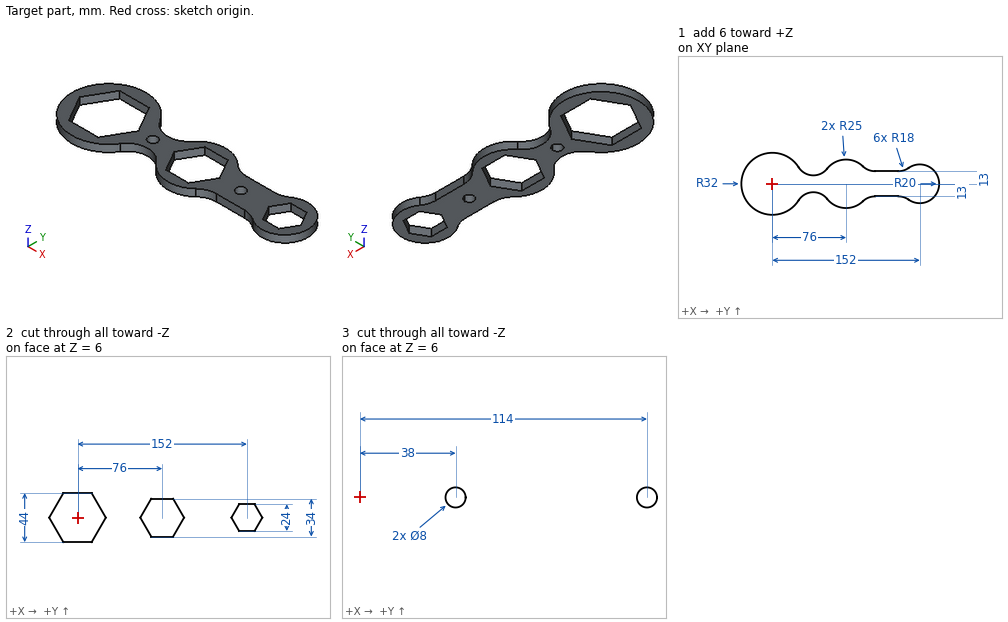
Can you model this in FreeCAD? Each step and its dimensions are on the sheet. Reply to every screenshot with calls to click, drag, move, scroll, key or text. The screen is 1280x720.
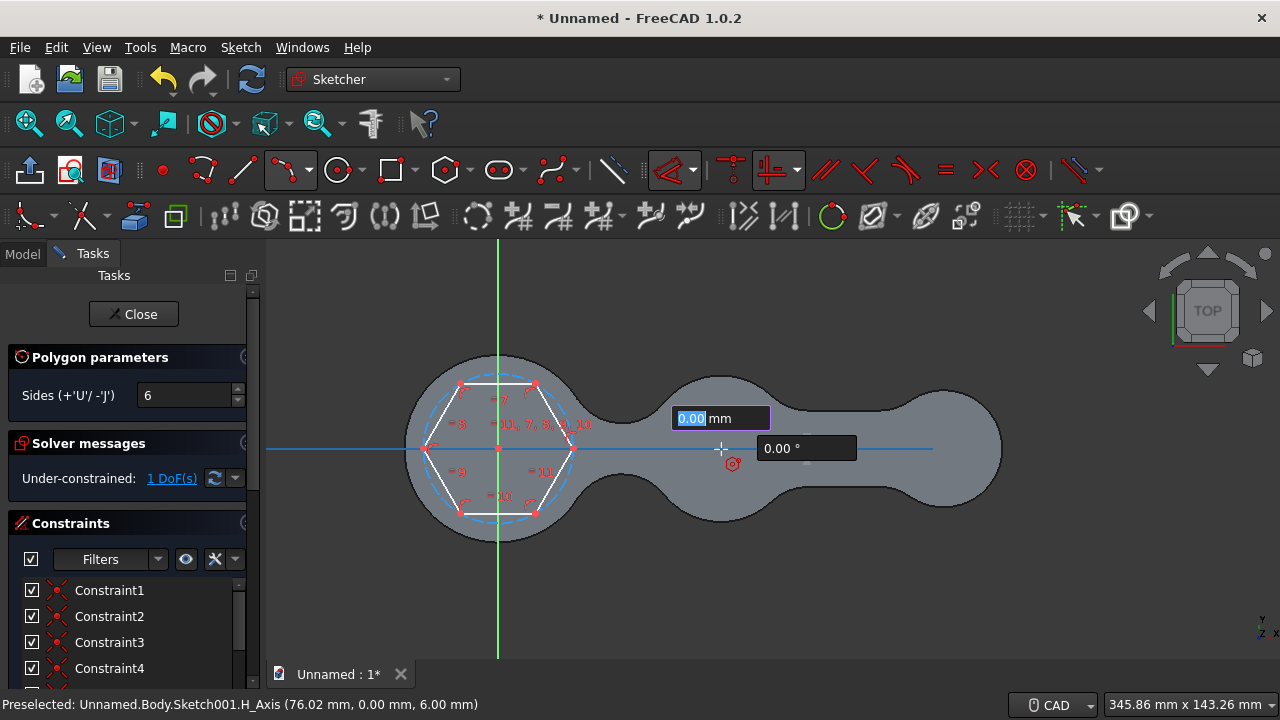
click(778, 449)
key(Escape)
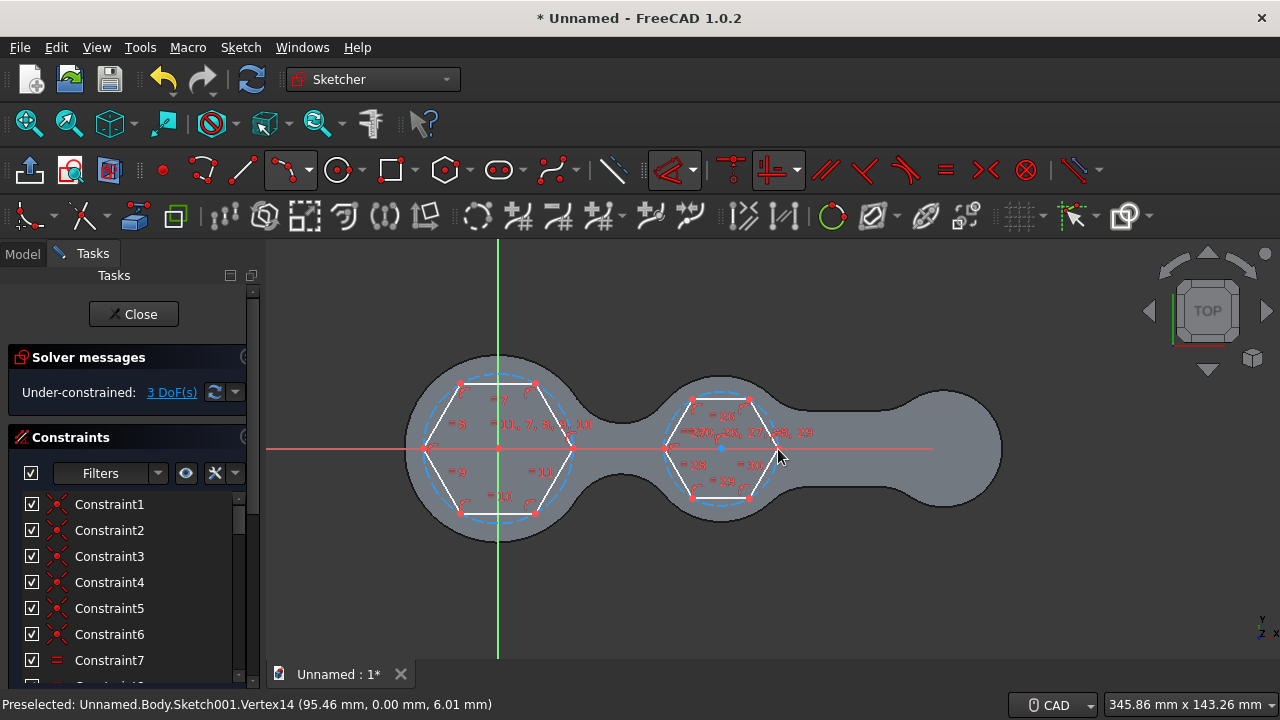
click(446, 170)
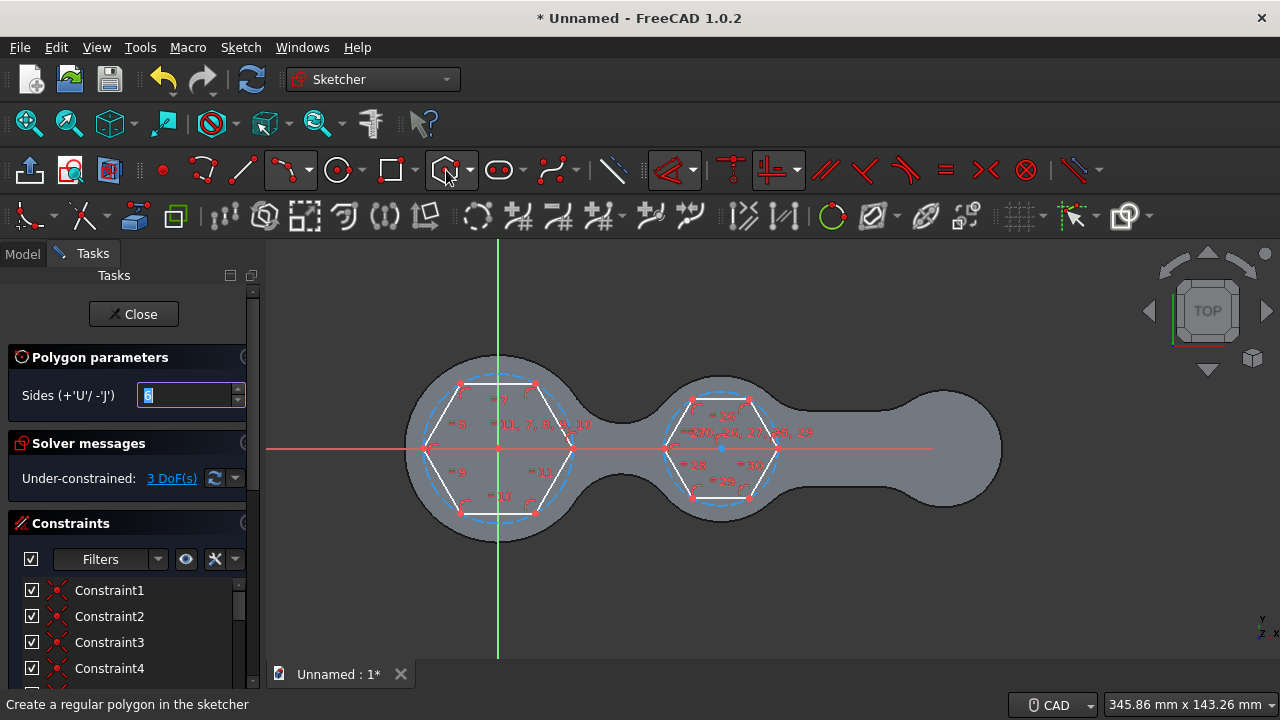
click(944, 449)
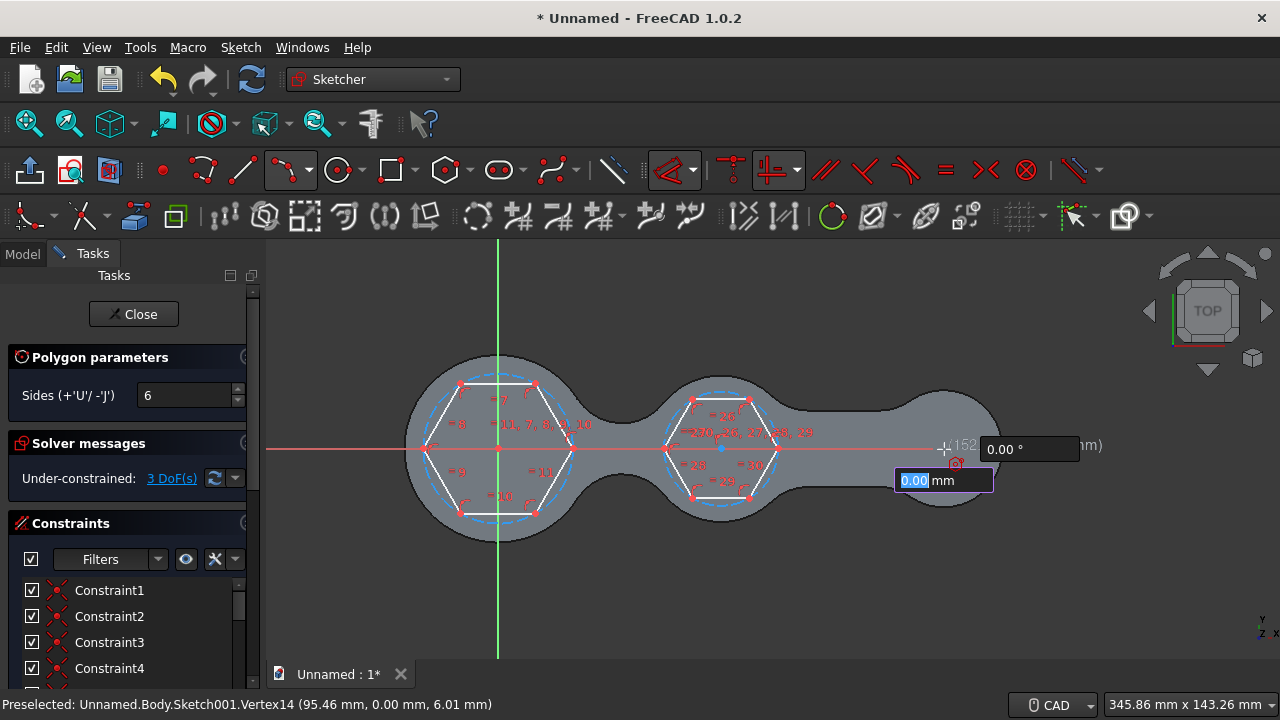
click(984, 449)
key(Escape)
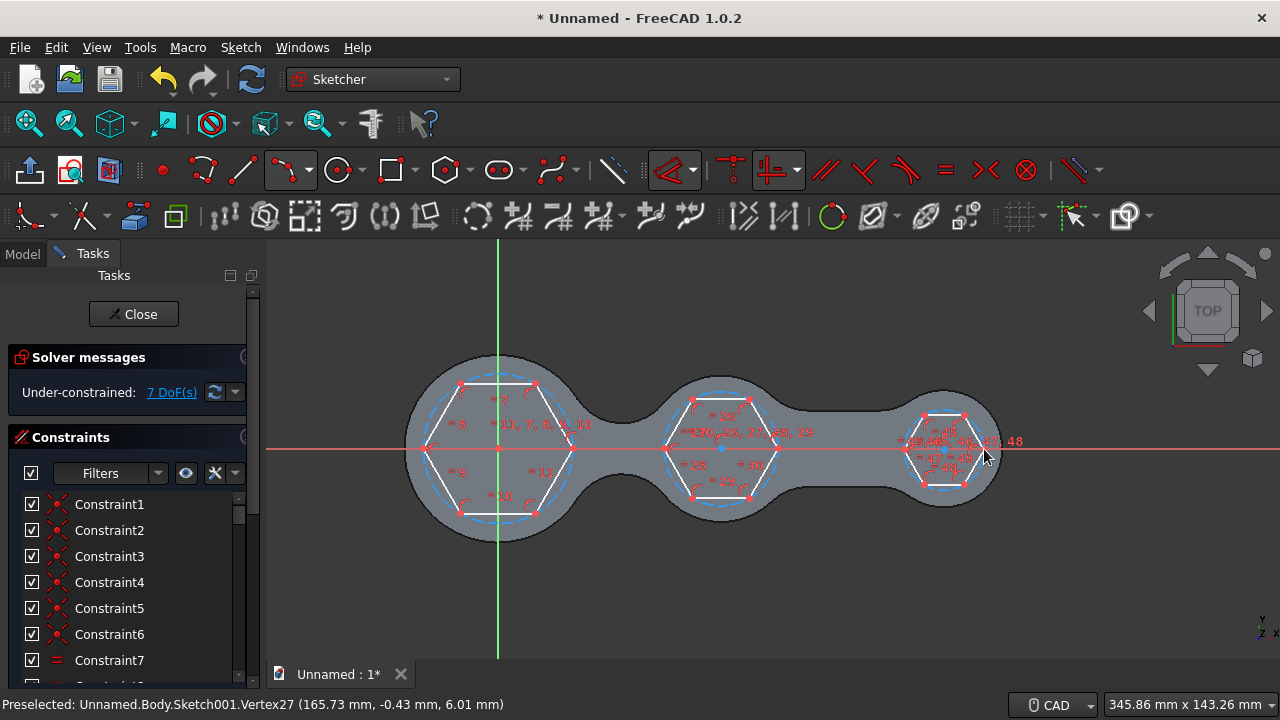
scroll(944, 415, up, 5)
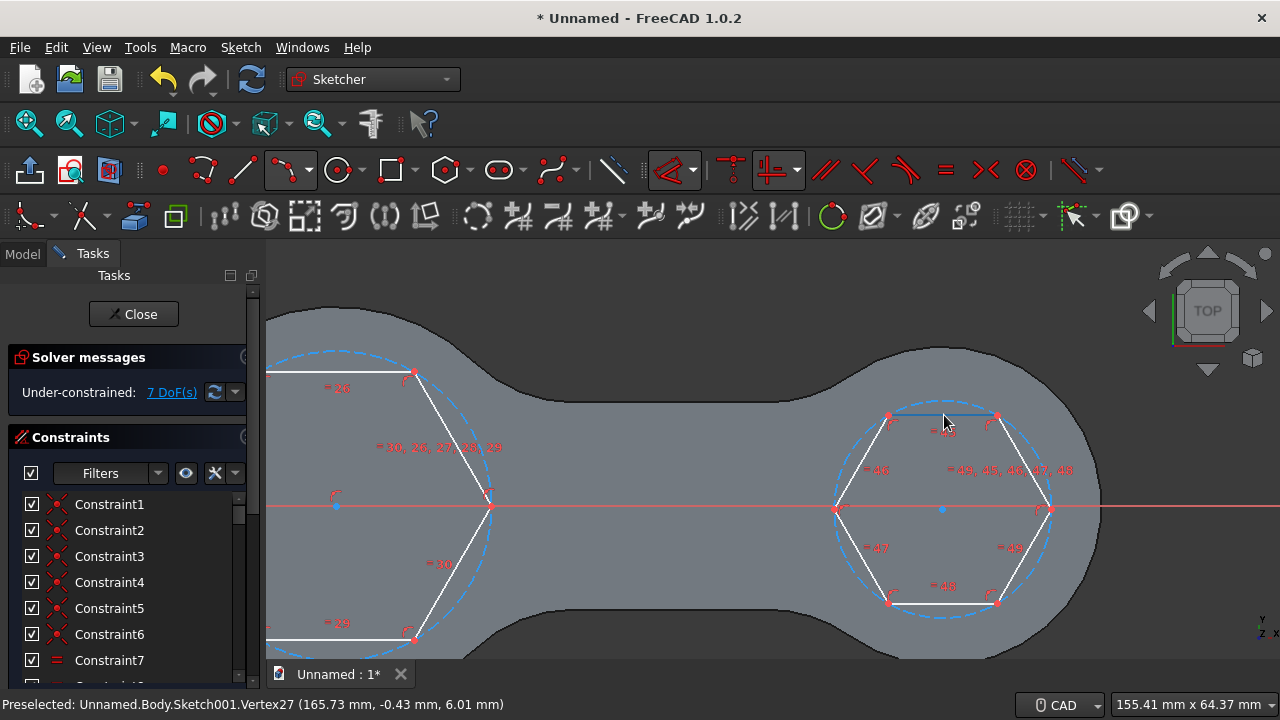
click(943, 415)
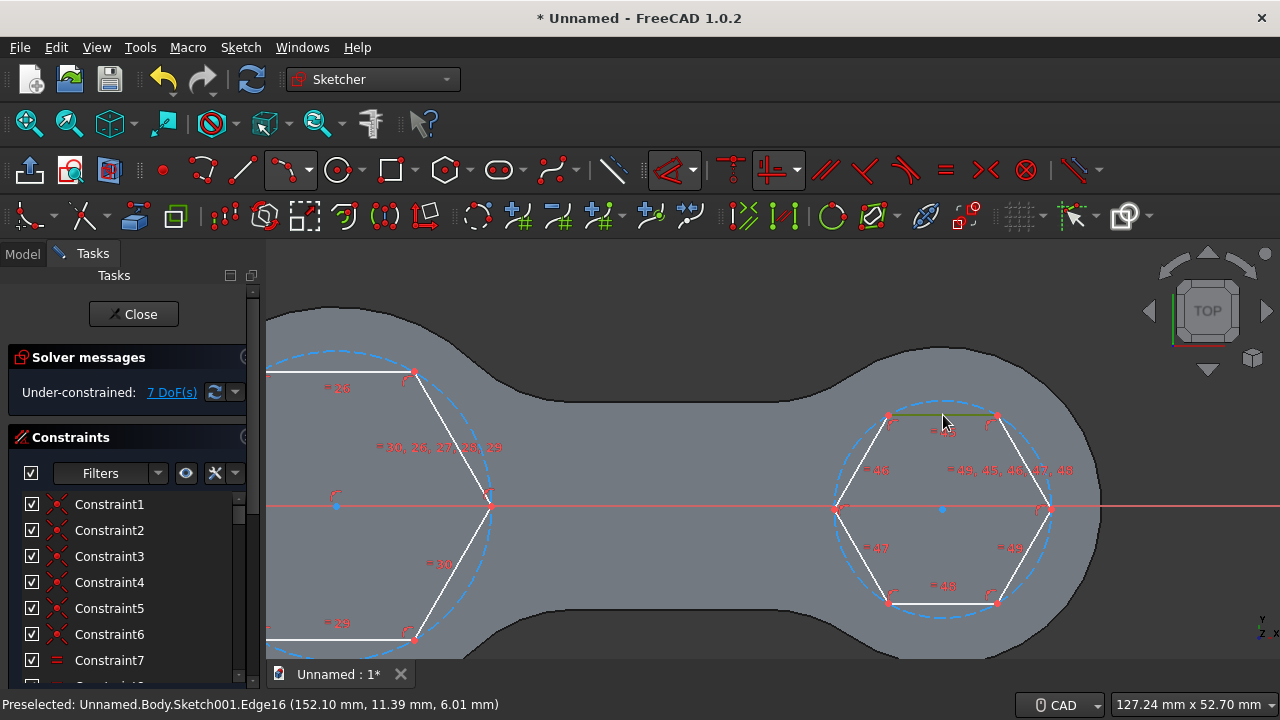
key(h)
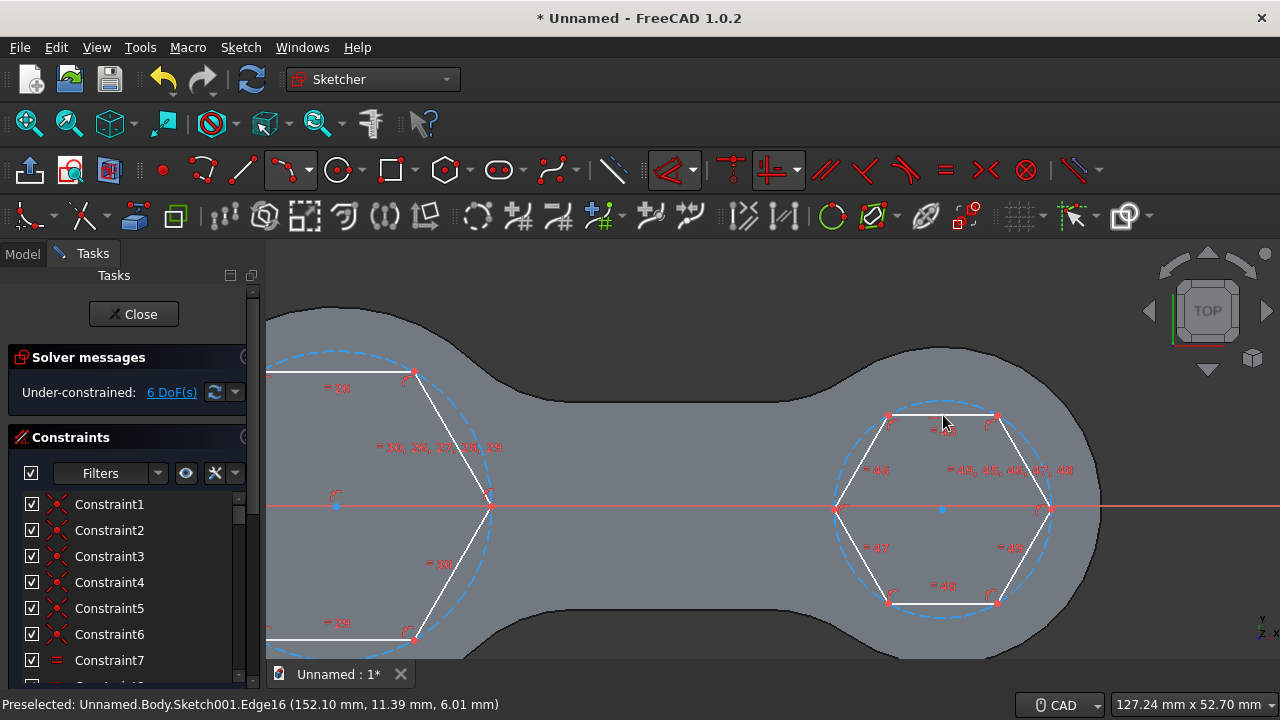
click(943, 509)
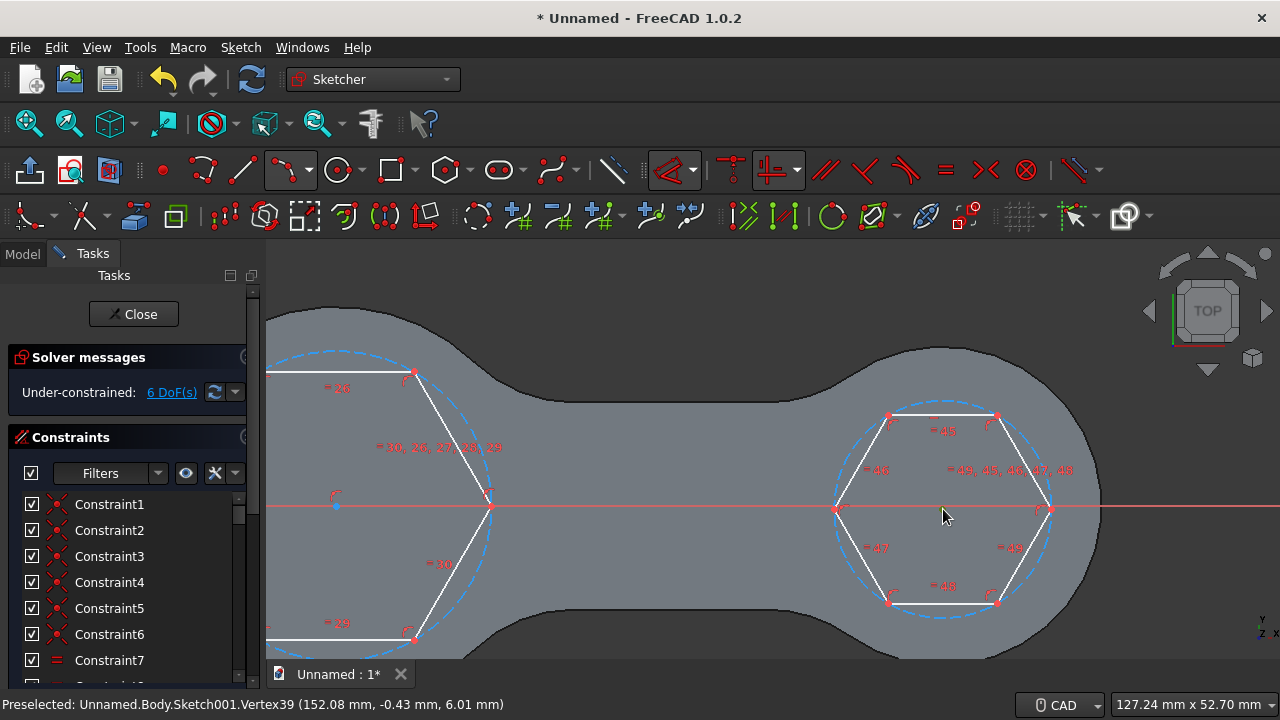
click(353, 506)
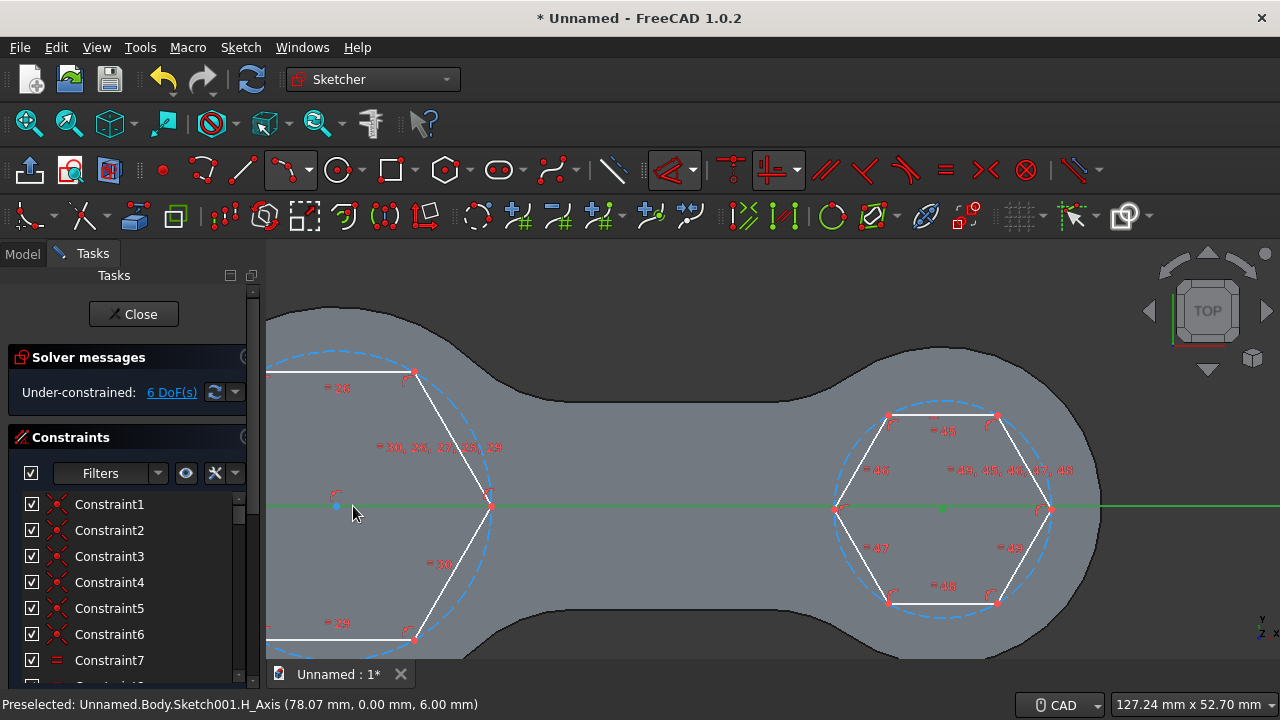
click(732, 170)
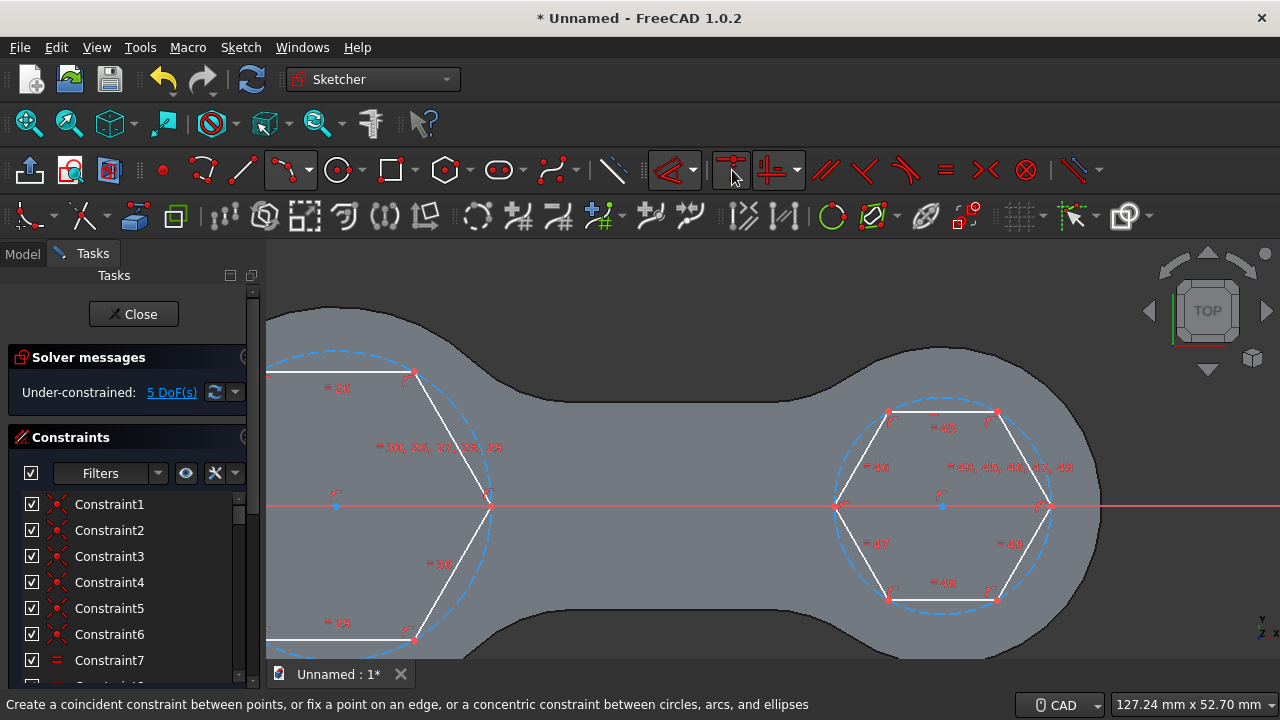
scroll(945, 416, down, 5)